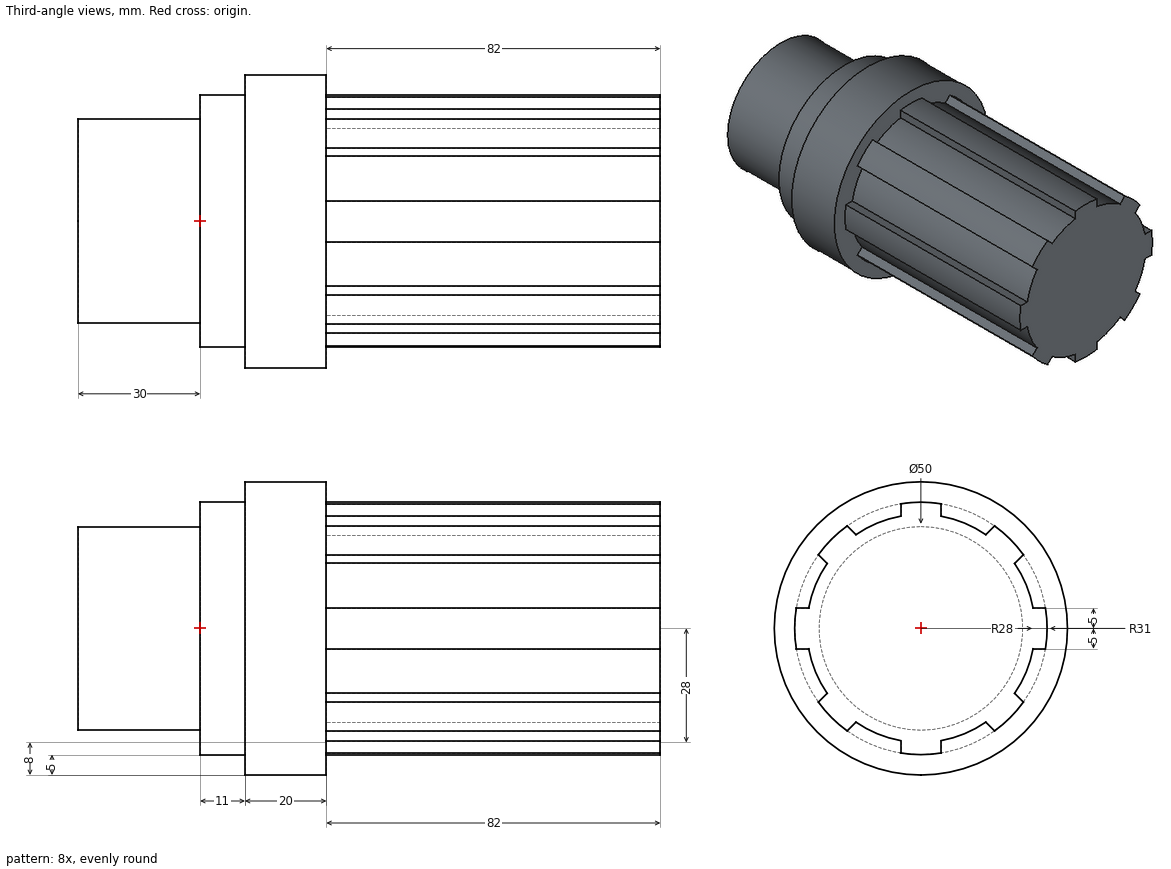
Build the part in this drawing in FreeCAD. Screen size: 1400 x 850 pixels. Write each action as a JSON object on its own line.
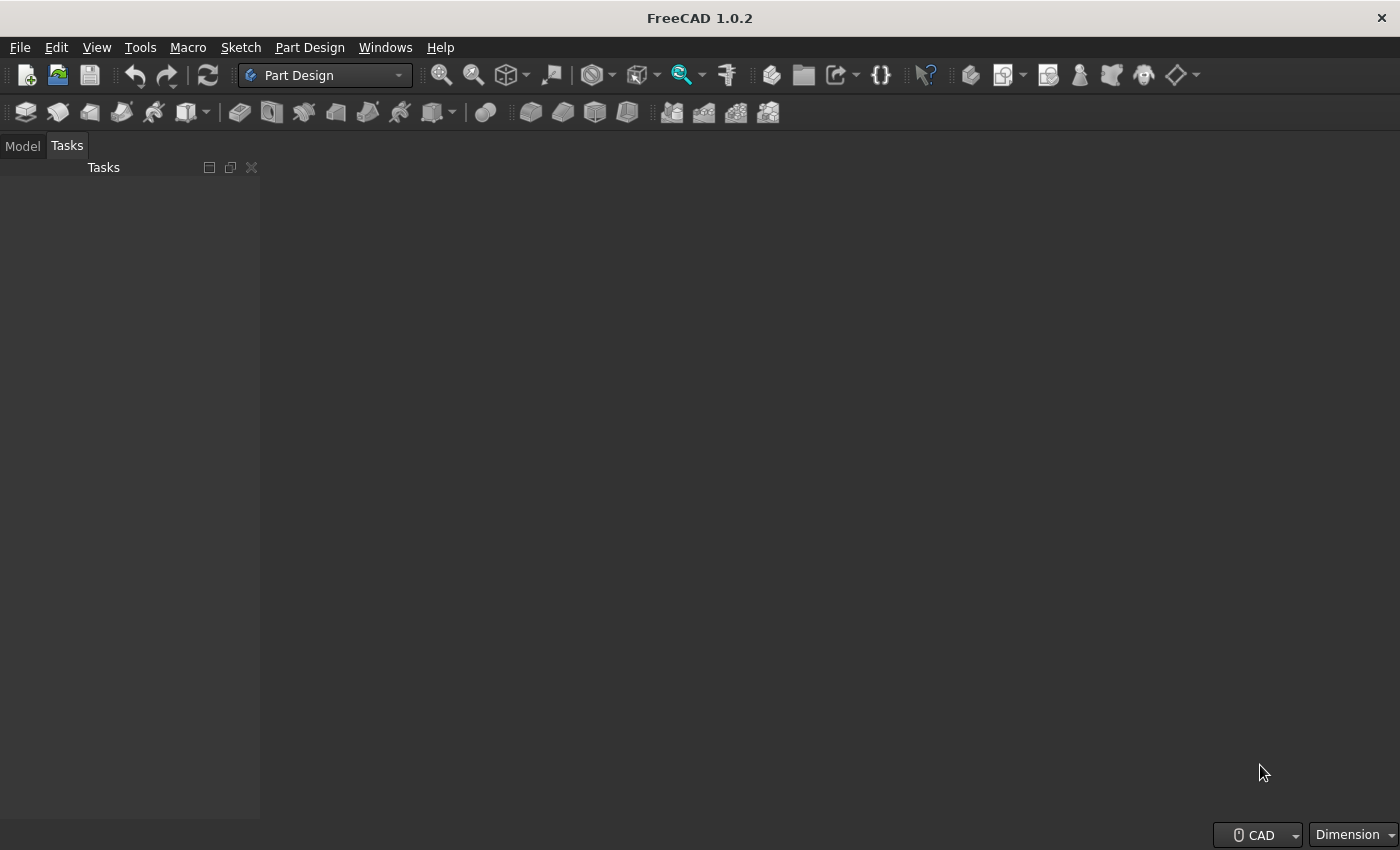
{"action": "left_click", "coordinate": [26, 76]}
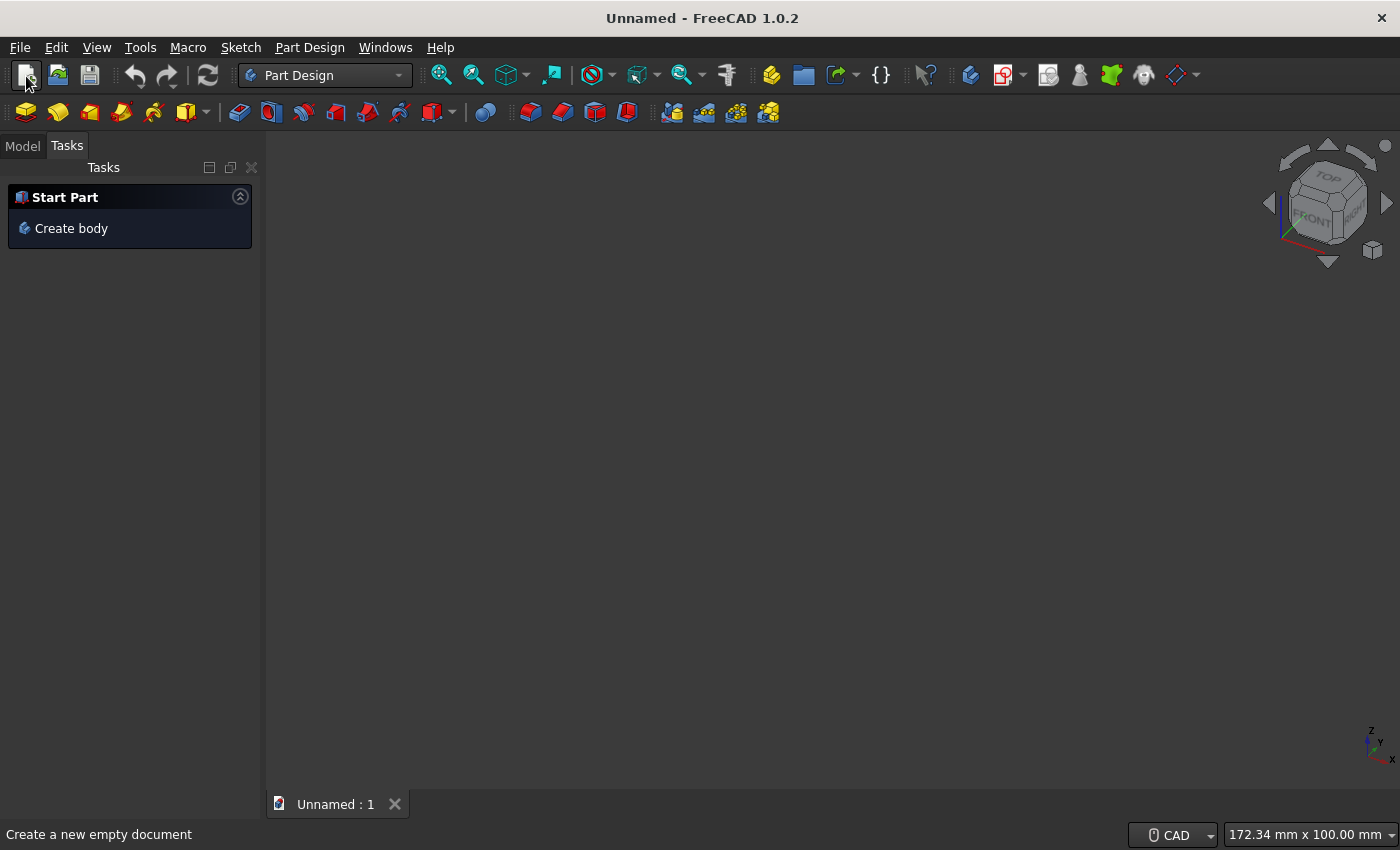
{"action": "left_click", "coordinate": [1004, 76]}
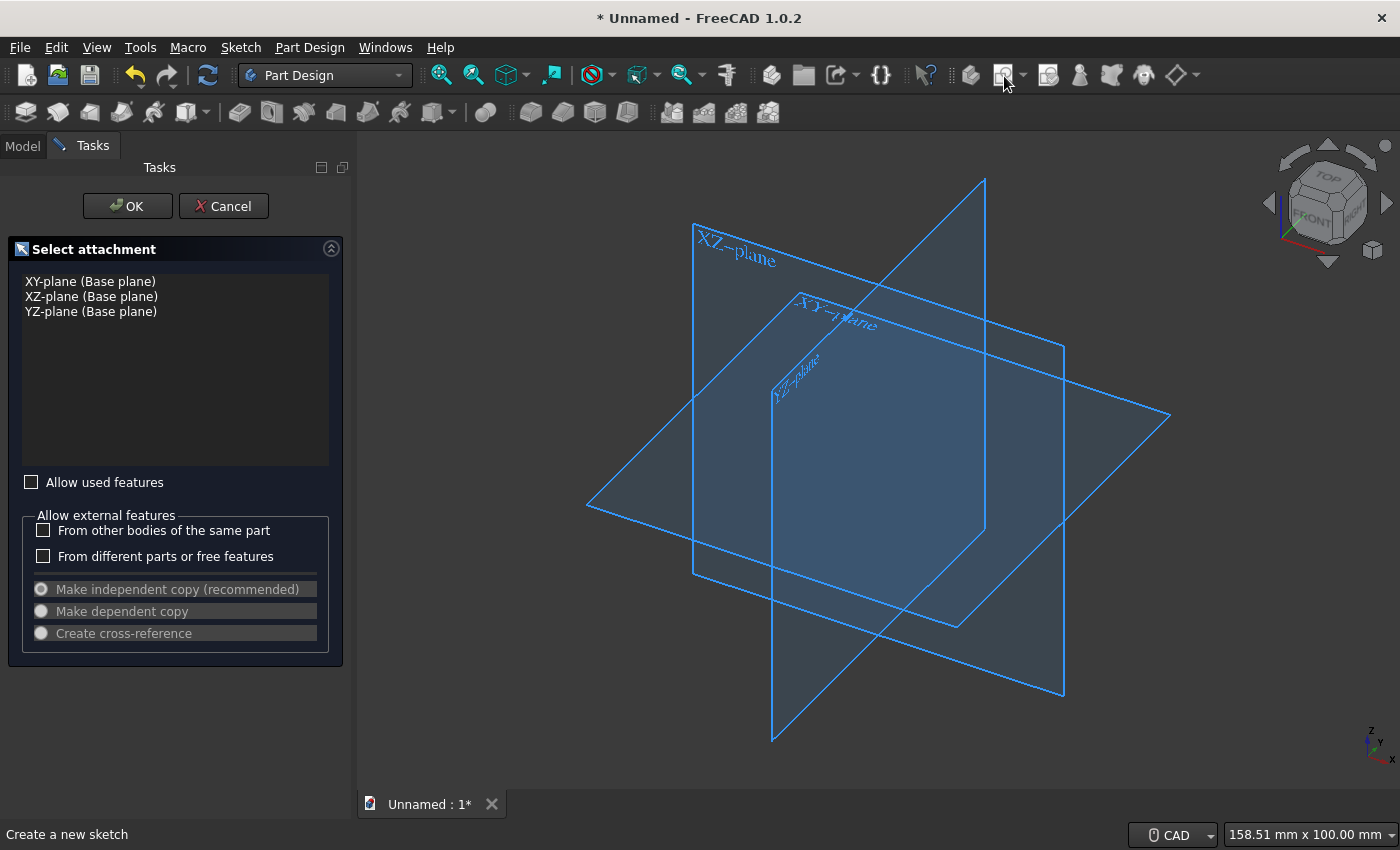
{"action": "left_click", "coordinate": [82, 296]}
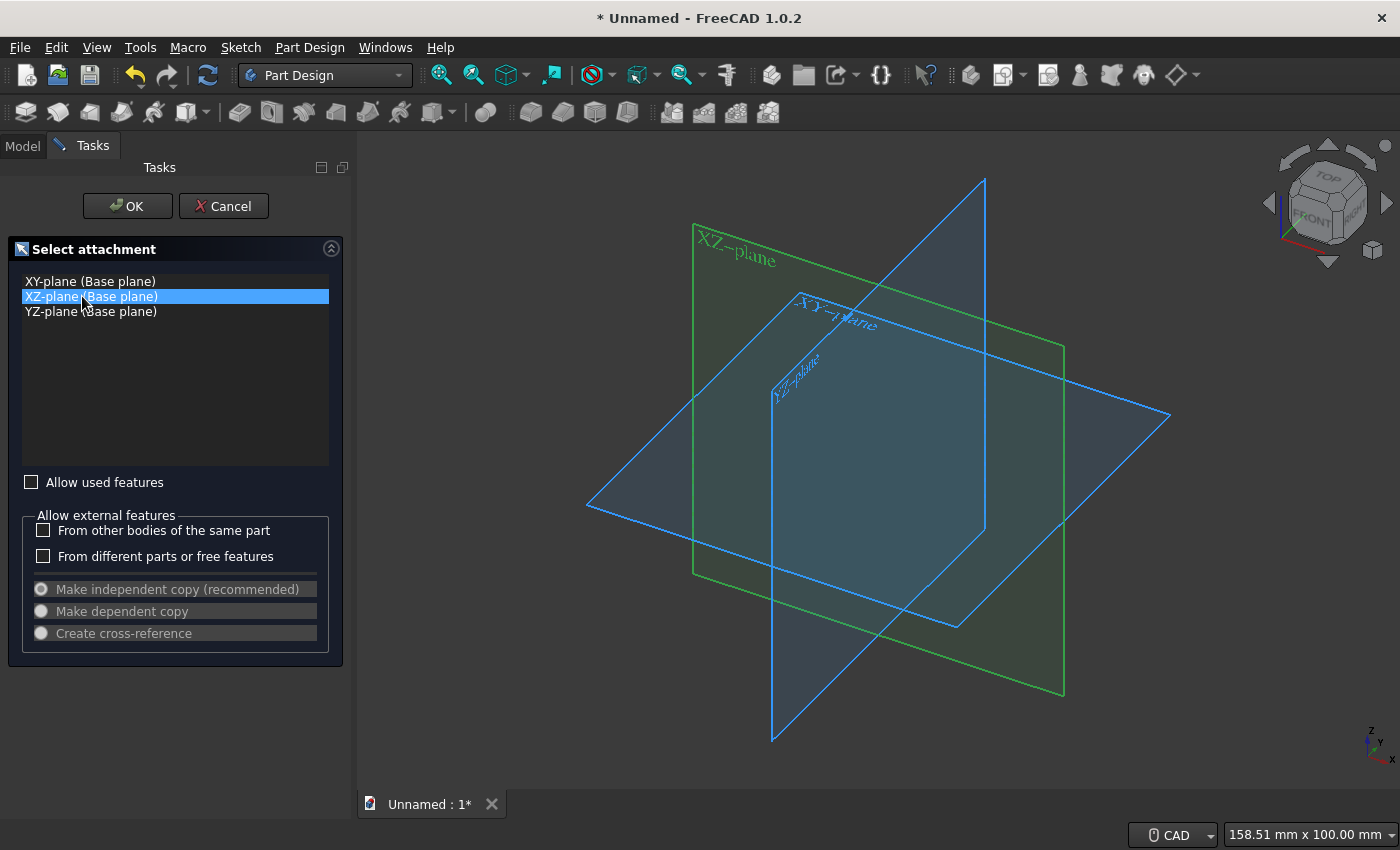
{"action": "left_click", "coordinate": [128, 206]}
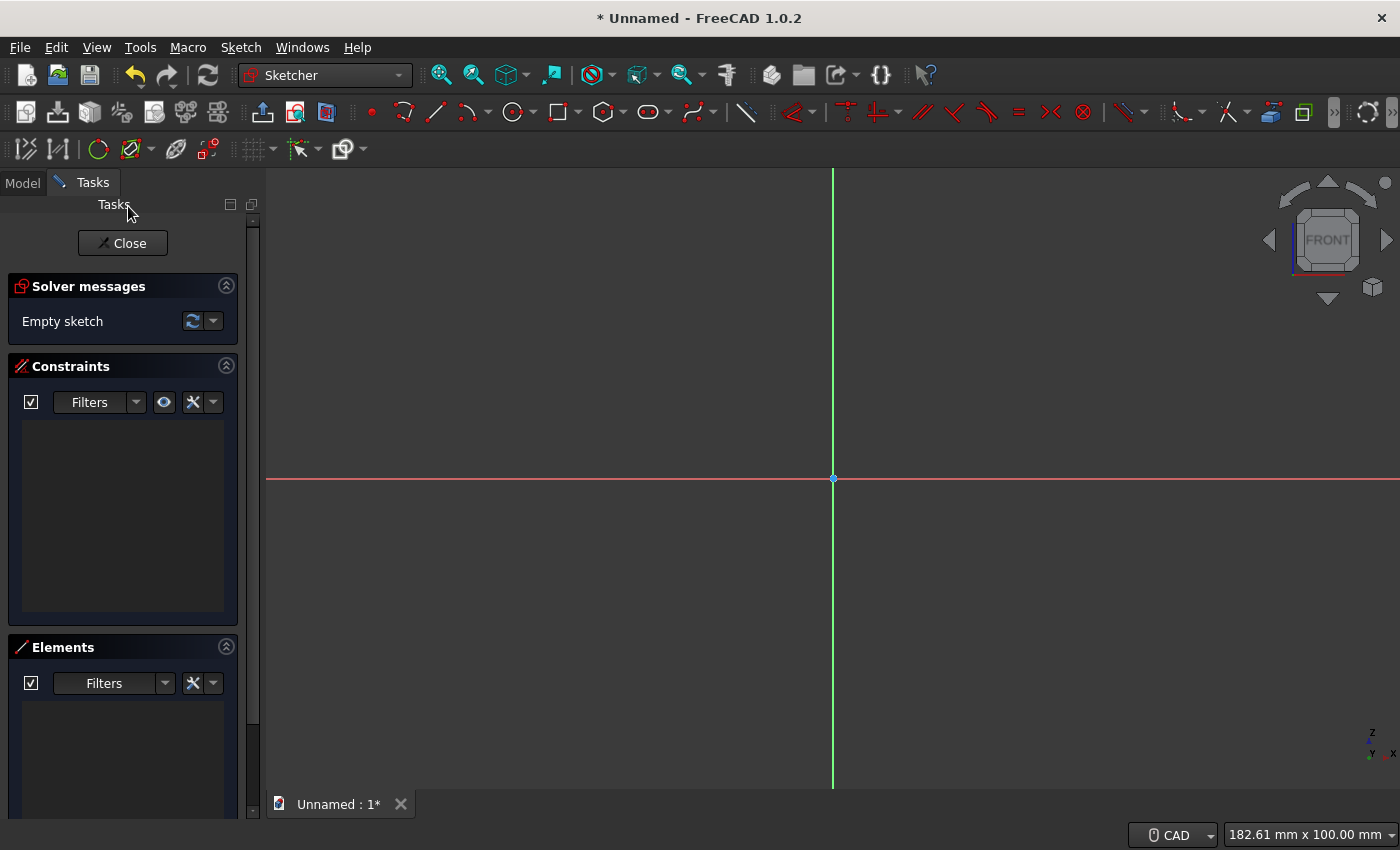
{"action": "scroll", "coordinate": [294, 251], "scroll_direction": "down", "scroll_amount": 2}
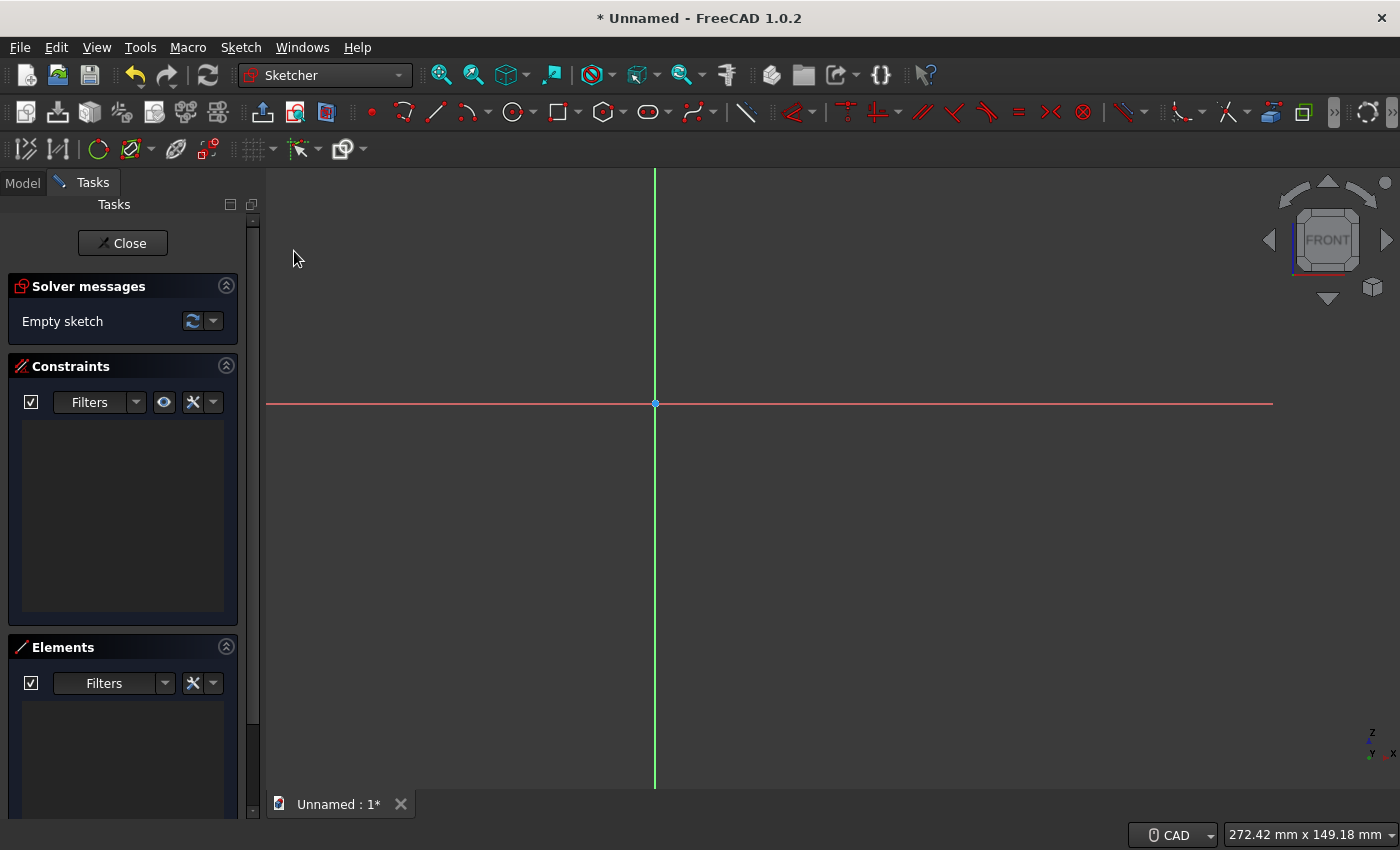
{"action": "scroll", "coordinate": [1147, 478], "scroll_direction": "up", "scroll_amount": 2}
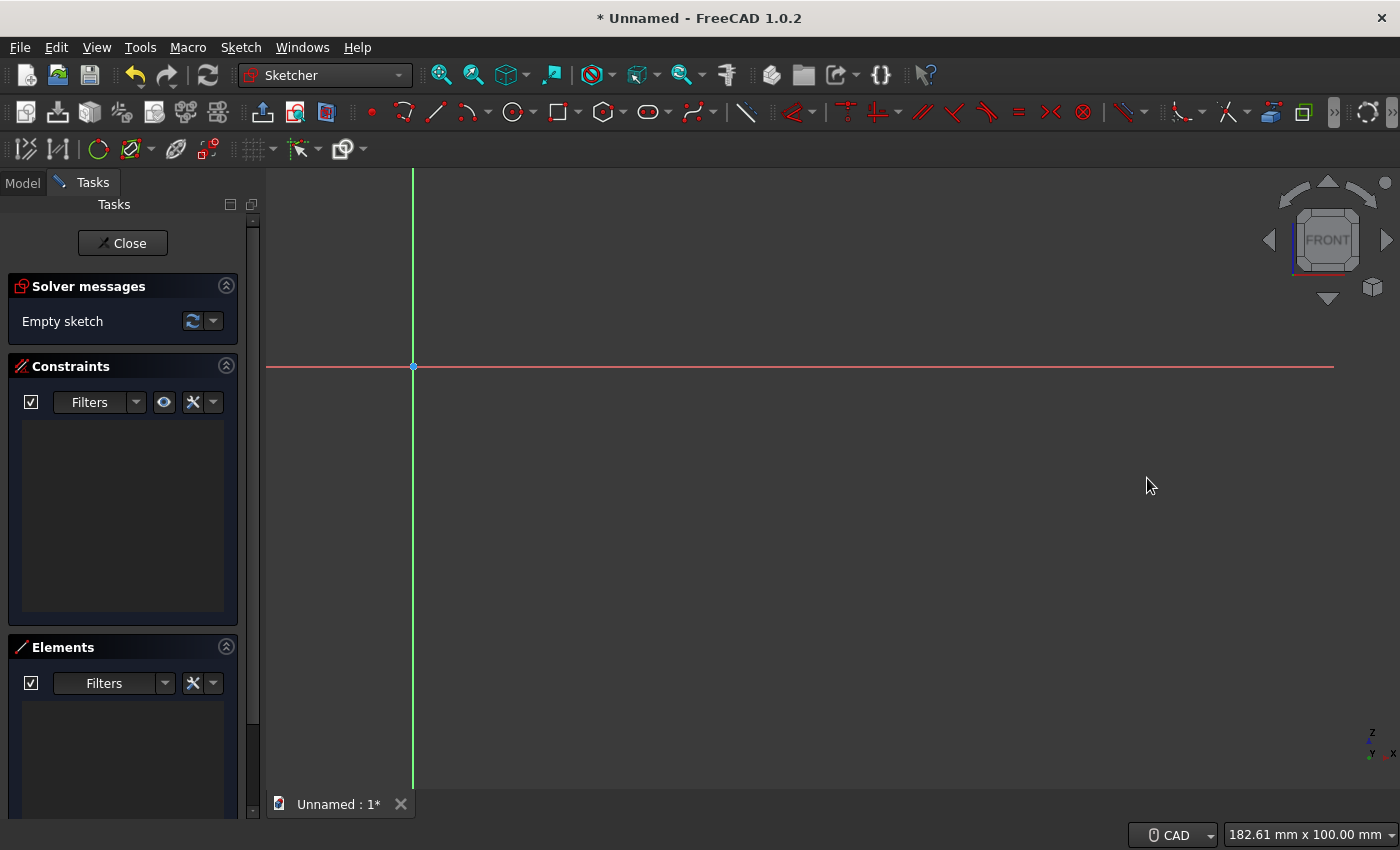
{"action": "left_click", "coordinate": [404, 112]}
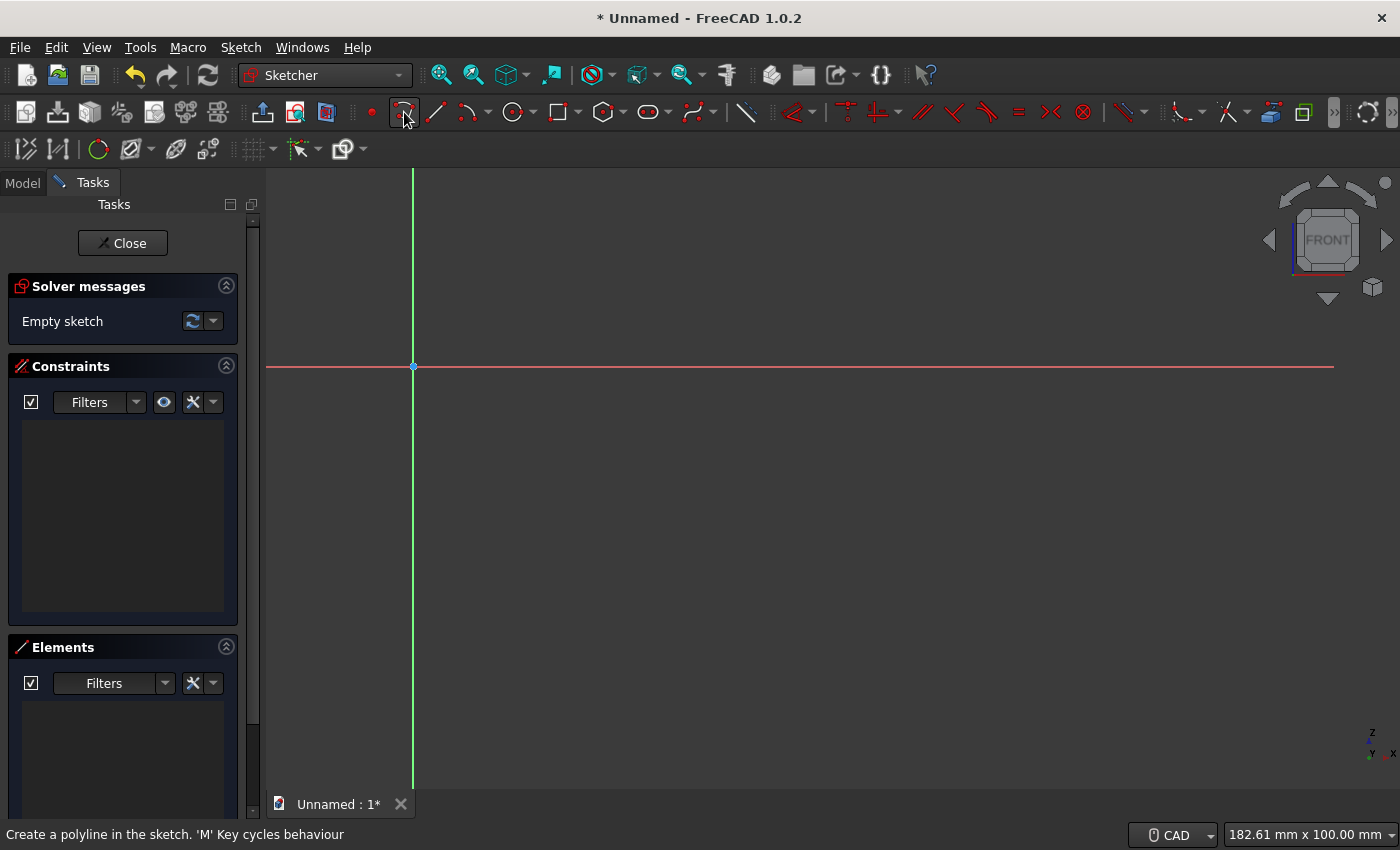
{"action": "left_click", "coordinate": [413, 367]}
{"action": "left_click", "coordinate": [1115, 376]}
{"action": "left_click", "coordinate": [1115, 541]}
{"action": "left_click", "coordinate": [606, 541]}
{"action": "left_click", "coordinate": [606, 590]}
{"action": "left_click", "coordinate": [481, 590]}
{"action": "left_click", "coordinate": [481, 559]}
{"action": "left_click", "coordinate": [422, 559]}
{"action": "left_click", "coordinate": [413, 367]}
{"action": "key", "text": "Escape"}
{"action": "key", "text": "Escape"}